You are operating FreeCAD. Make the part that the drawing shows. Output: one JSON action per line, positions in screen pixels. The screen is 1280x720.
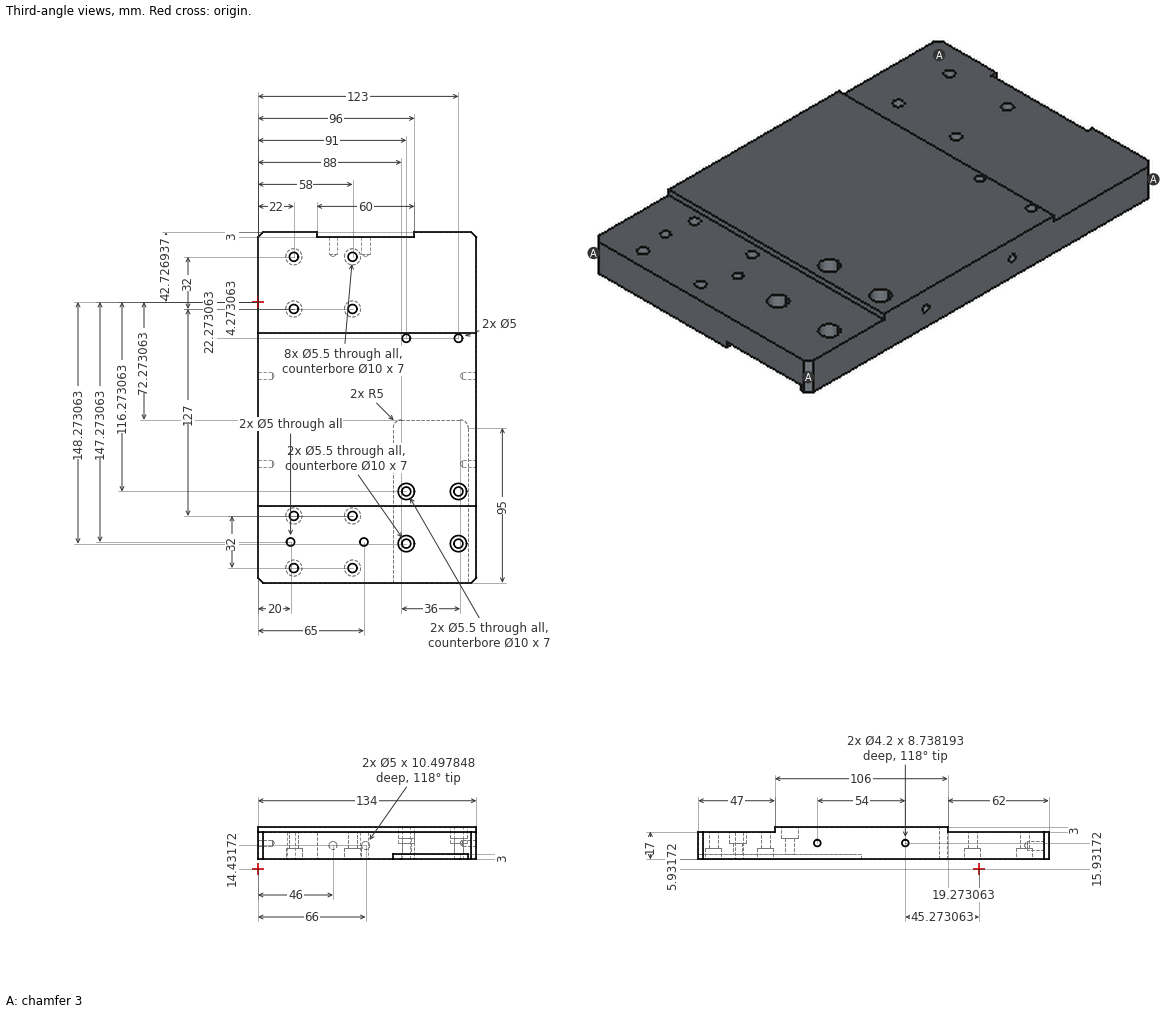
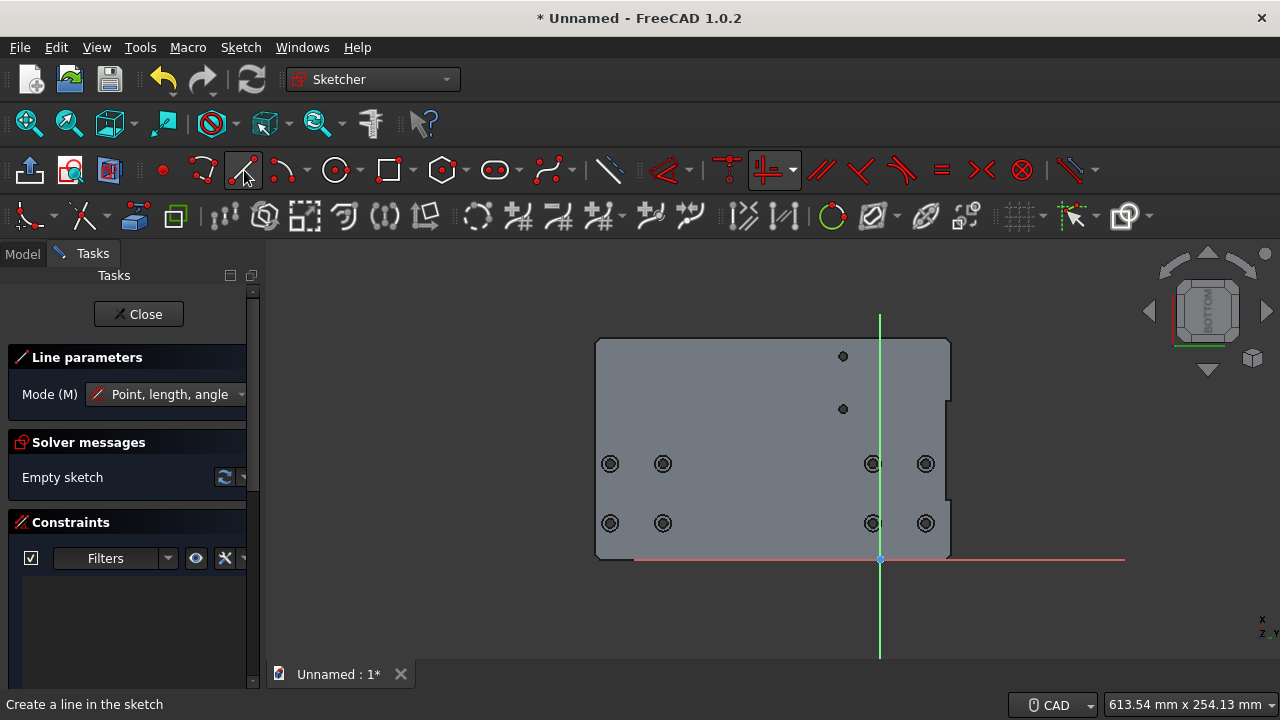
{"action": "left_click", "coordinate": [761, 414]}
{"action": "left_click", "coordinate": [761, 355]}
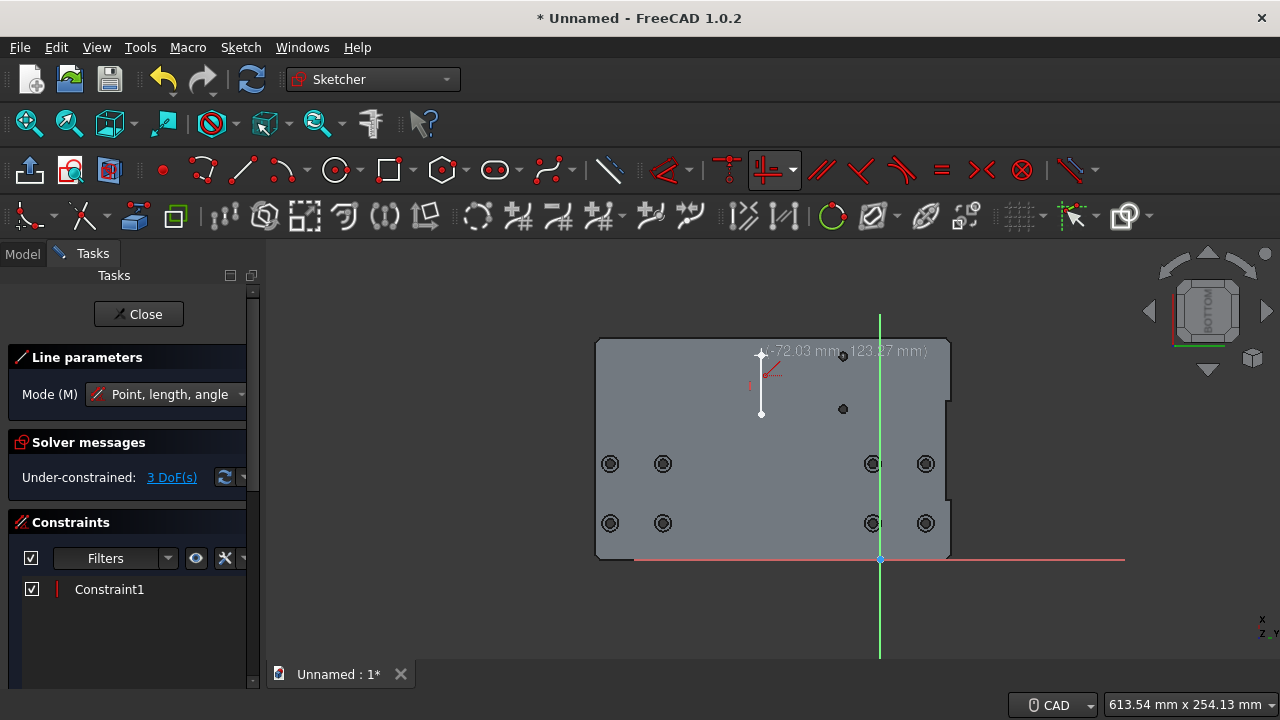
{"action": "left_click", "coordinate": [204, 170]}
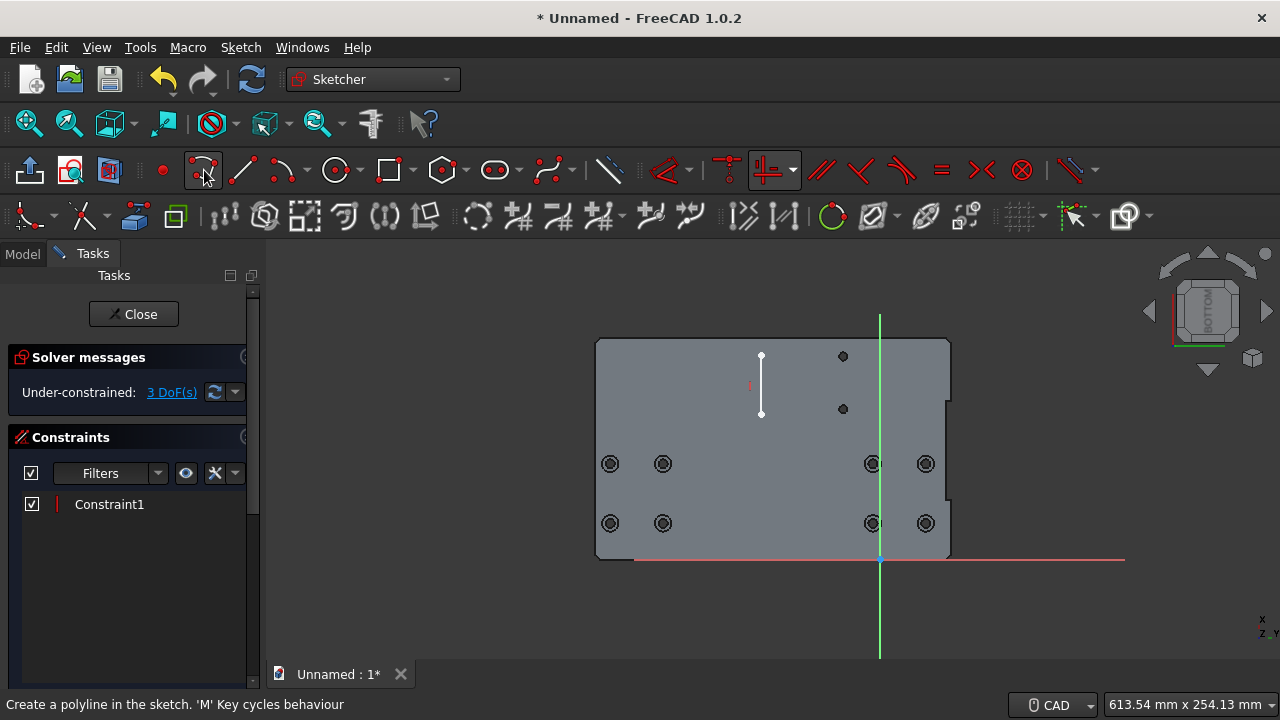
{"action": "scroll", "coordinate": [752, 347], "scroll_direction": "up", "scroll_amount": 2}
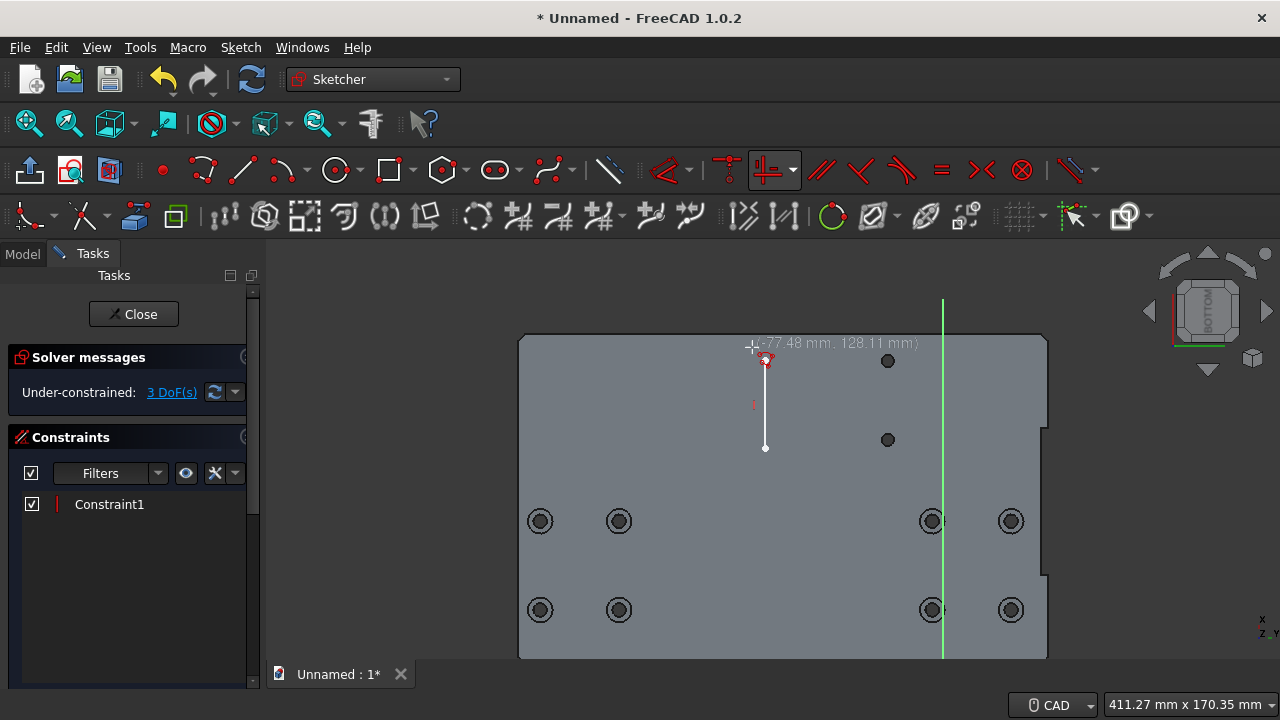
{"action": "left_click", "coordinate": [752, 346]}
{"action": "left_click", "coordinate": [518, 346]}
{"action": "left_click", "coordinate": [518, 460]}
{"action": "left_click", "coordinate": [752, 460]}
{"action": "right_click", "coordinate": [752, 460]}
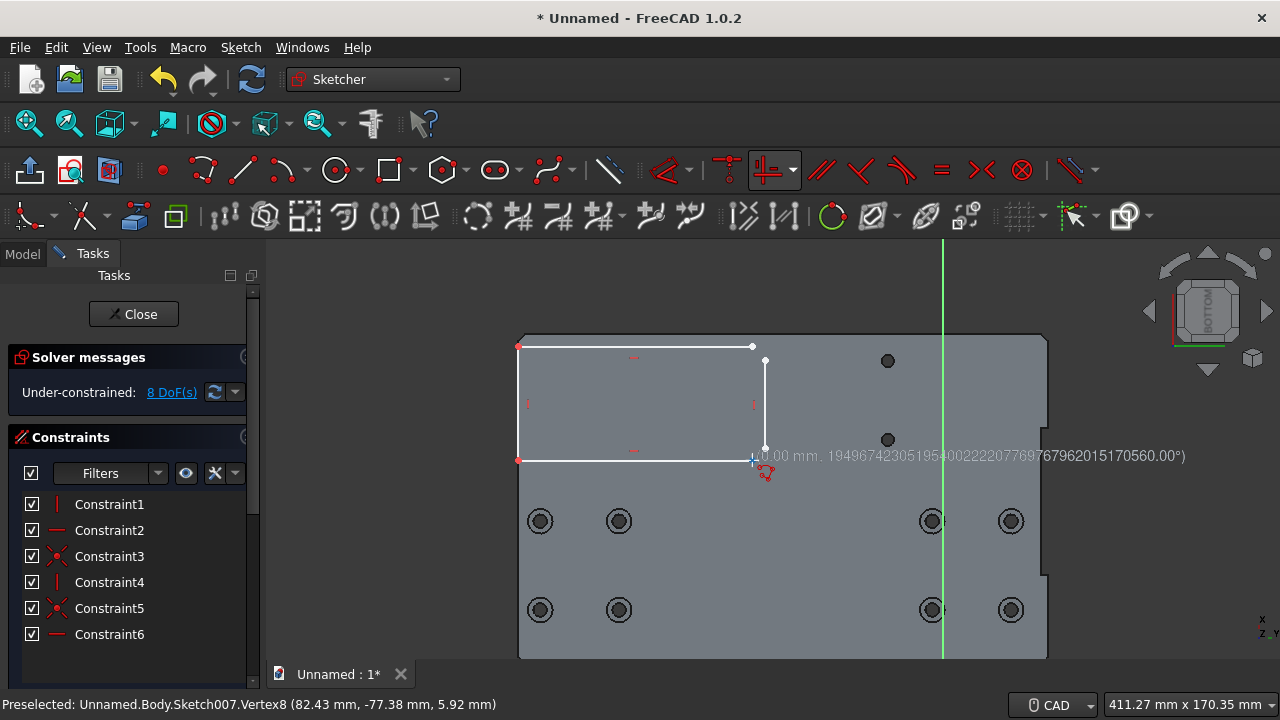
{"action": "left_click", "coordinate": [310, 170]}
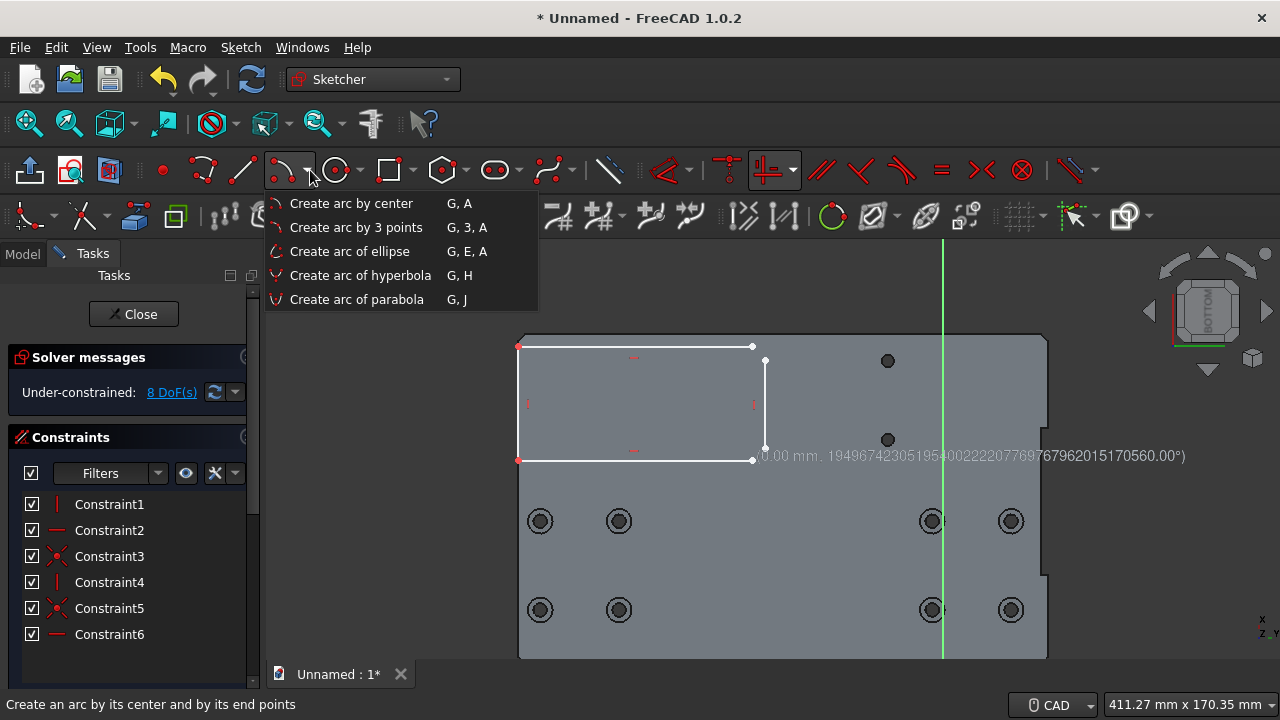
{"action": "left_click", "coordinate": [402, 227]}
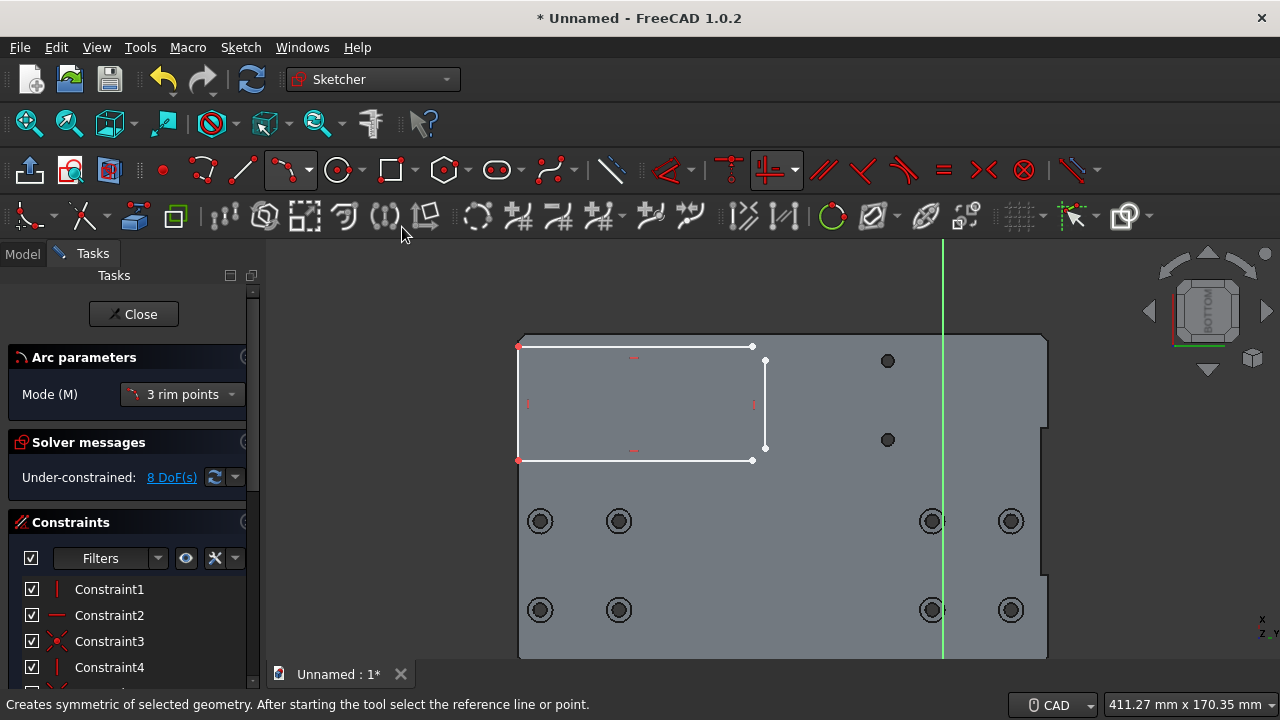
{"action": "left_click", "coordinate": [765, 360]}
{"action": "left_click", "coordinate": [752, 347]}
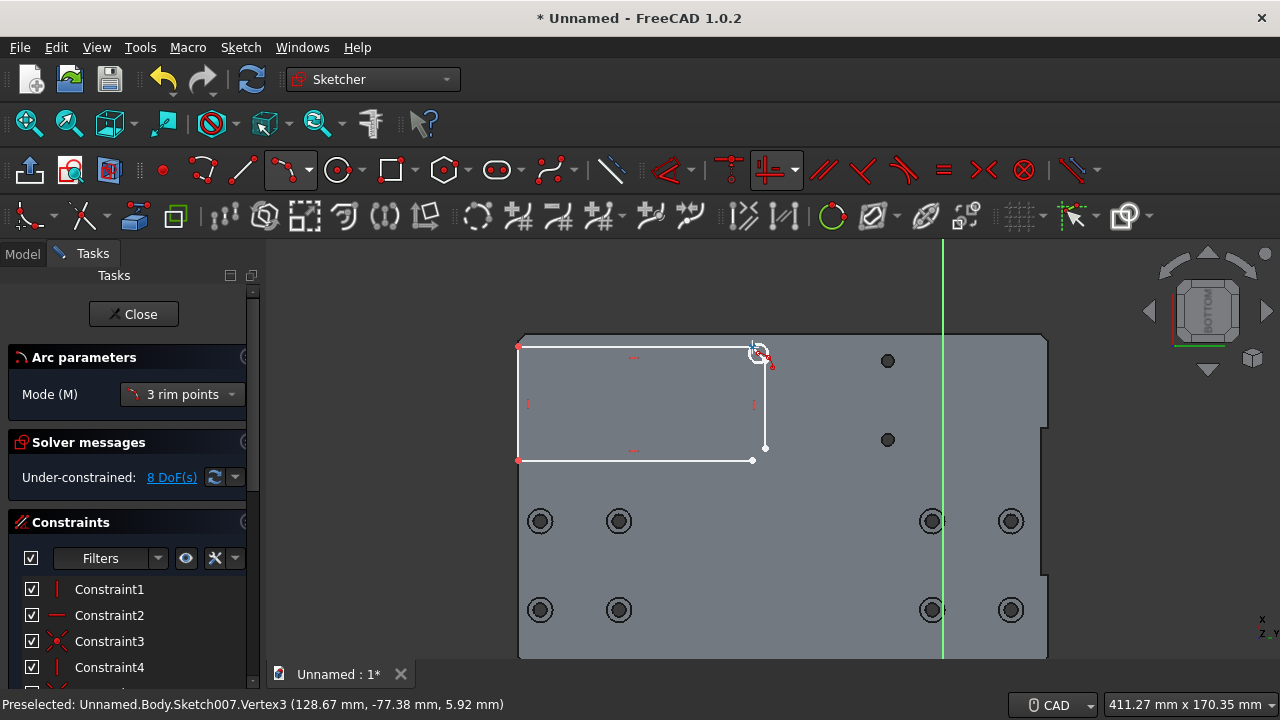
{"action": "scroll", "coordinate": [761, 350], "scroll_direction": "up", "scroll_amount": 8}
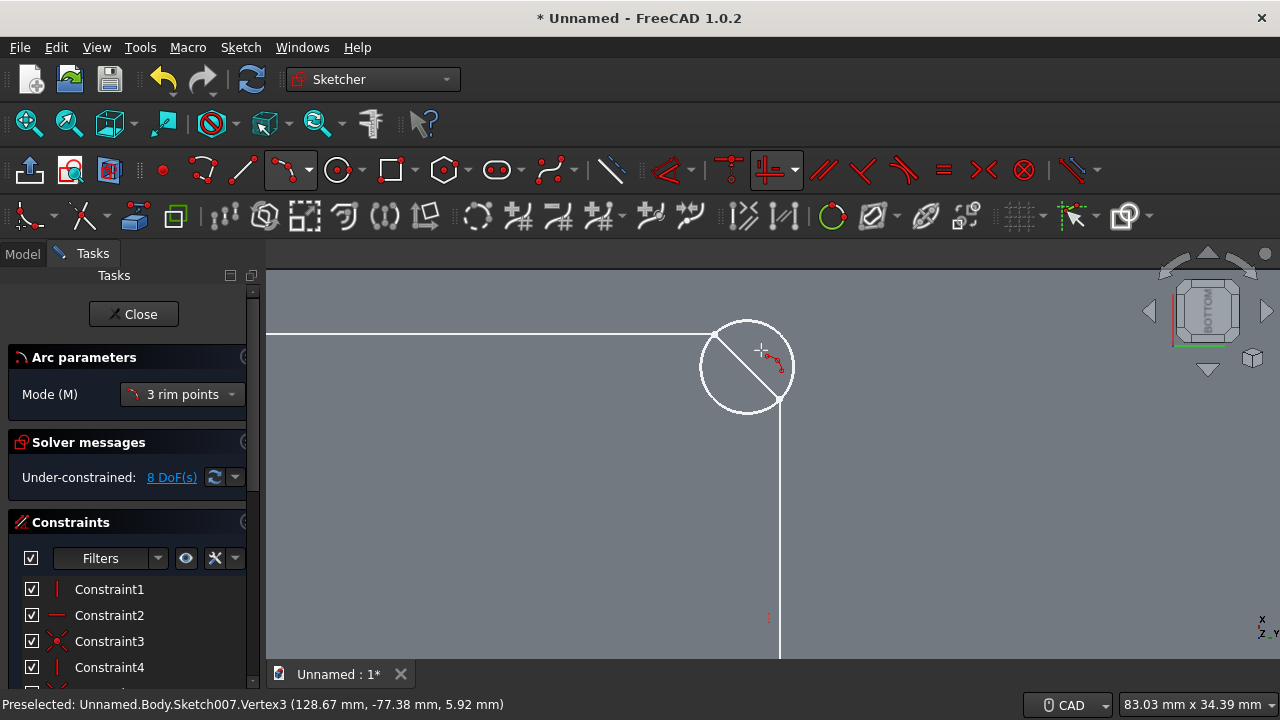
{"action": "left_click", "coordinate": [759, 348]}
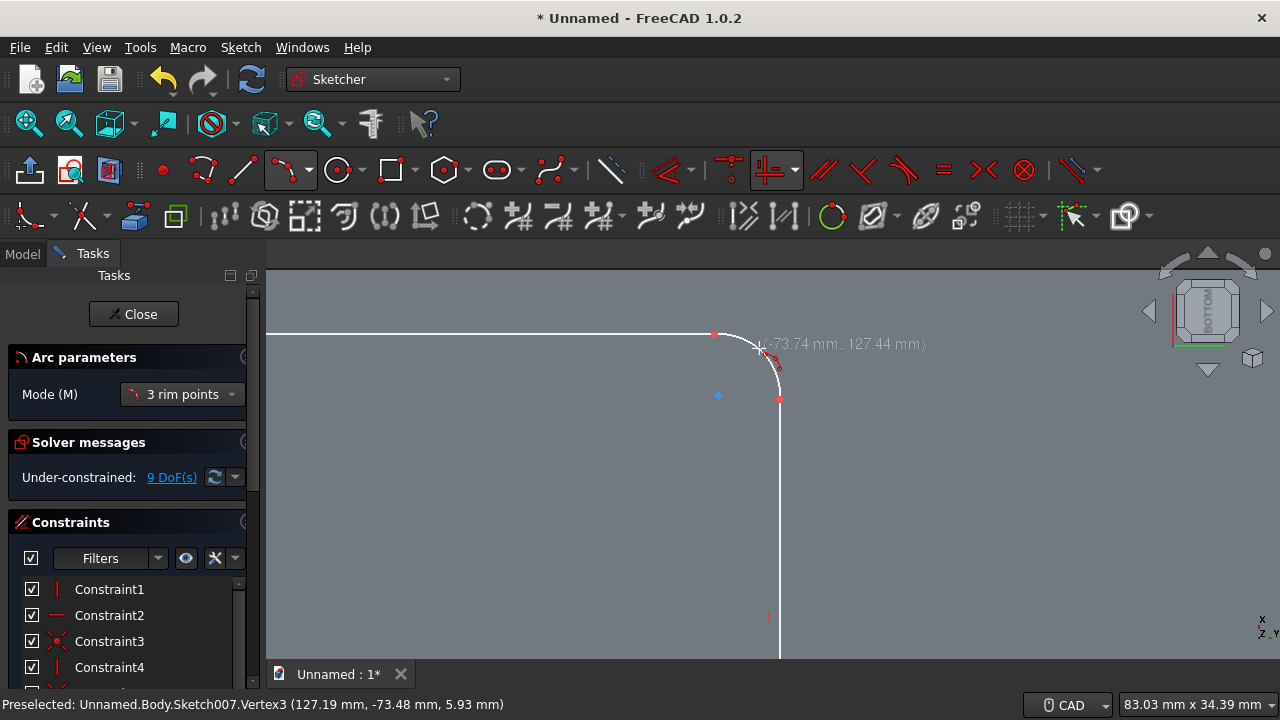
{"action": "scroll", "coordinate": [724, 317], "scroll_direction": "down", "scroll_amount": 9}